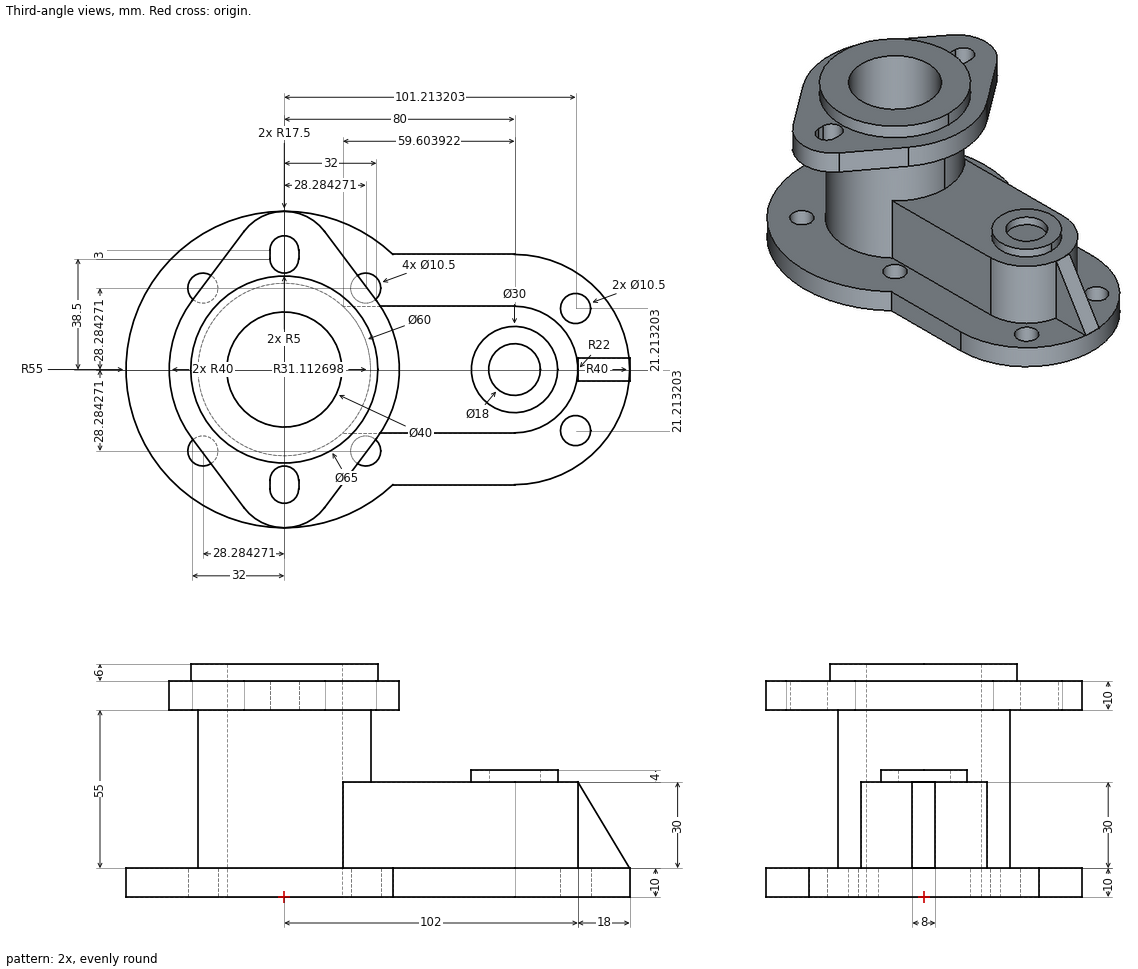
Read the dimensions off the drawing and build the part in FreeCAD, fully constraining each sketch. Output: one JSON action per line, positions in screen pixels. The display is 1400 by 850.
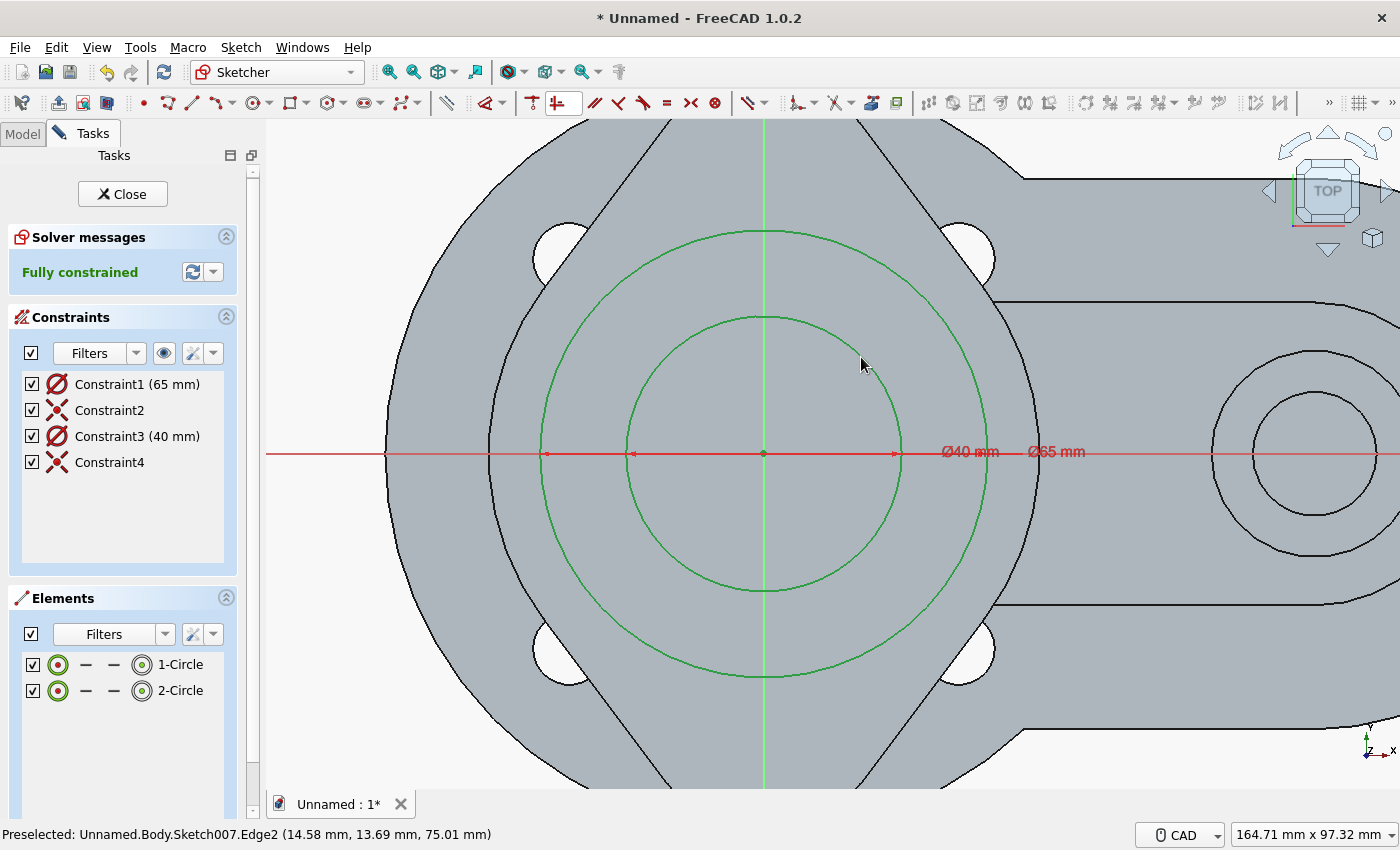
{"action": "left_click", "coordinate": [123, 194]}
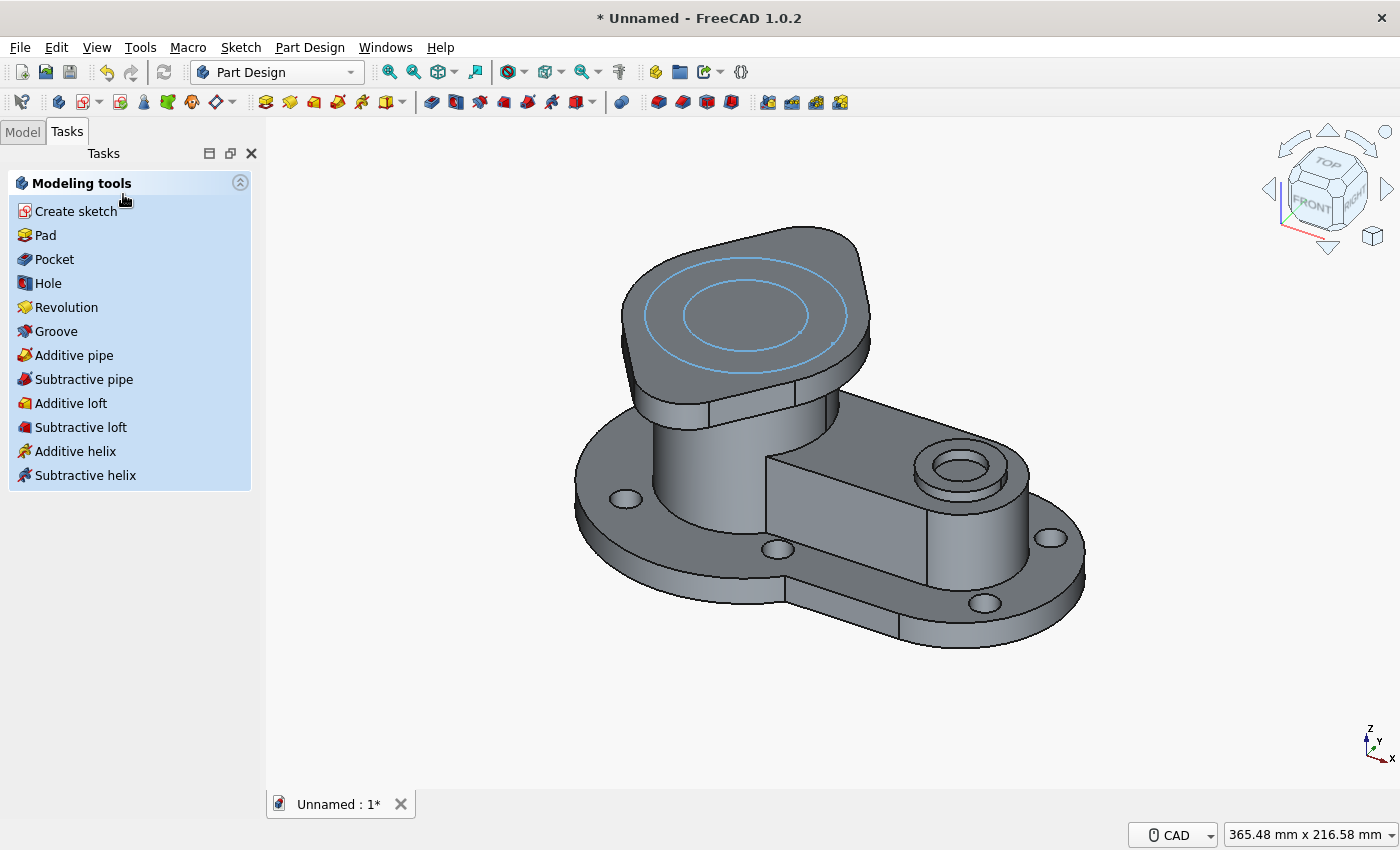
{"action": "left_click", "coordinate": [266, 102]}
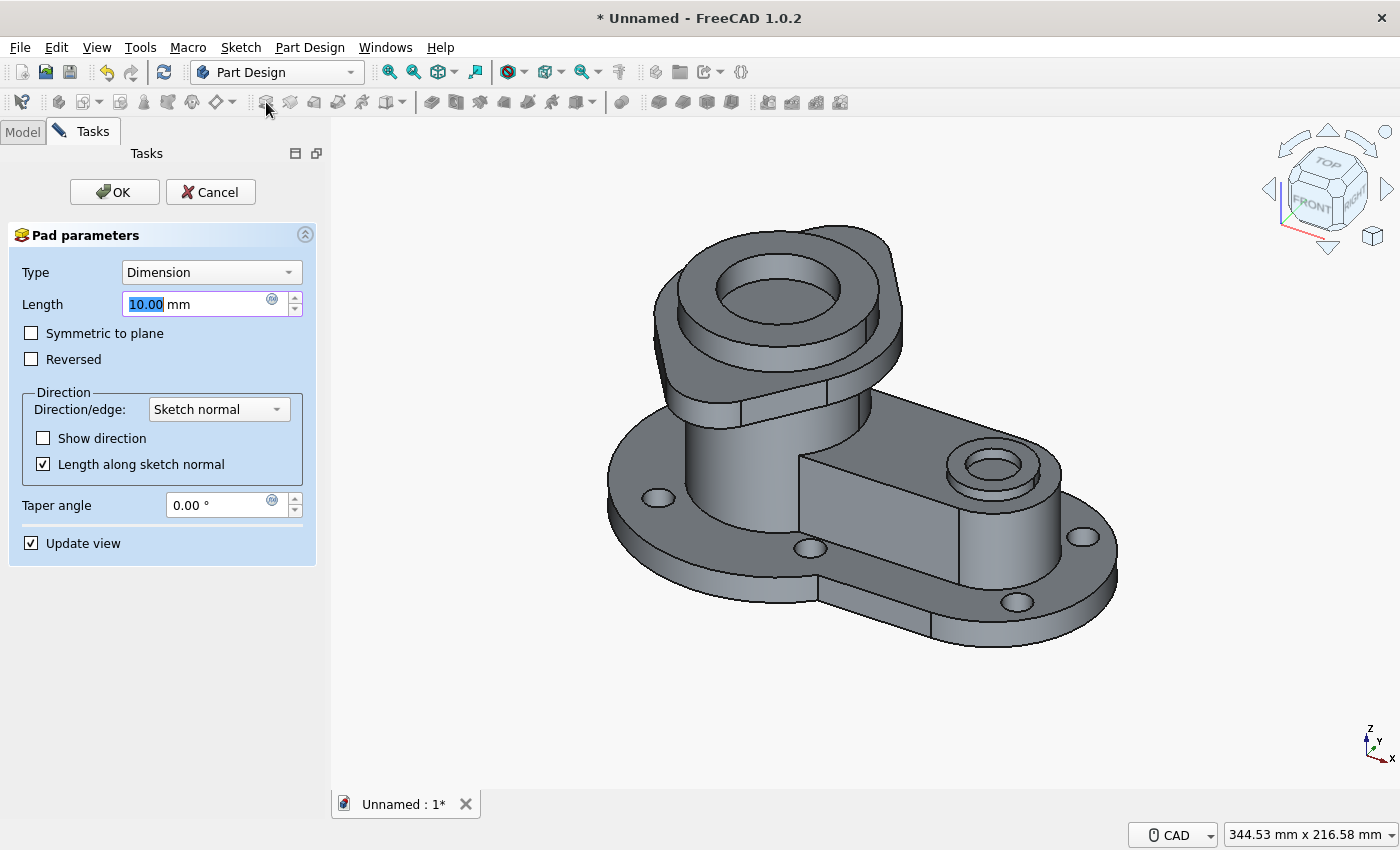
{"action": "type", "text": "6"}
{"action": "key", "text": "Tab"}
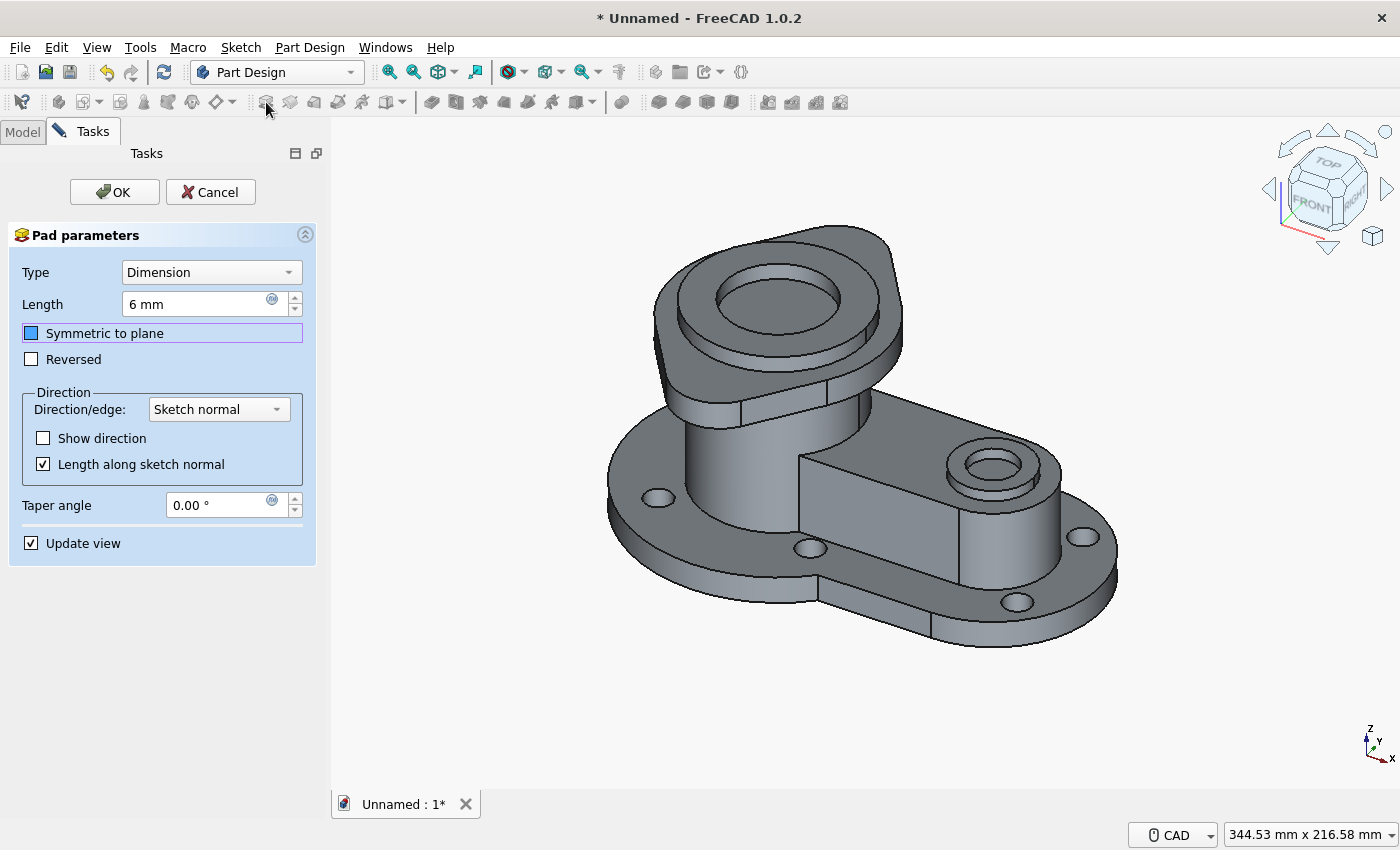
{"action": "left_click", "coordinate": [115, 192]}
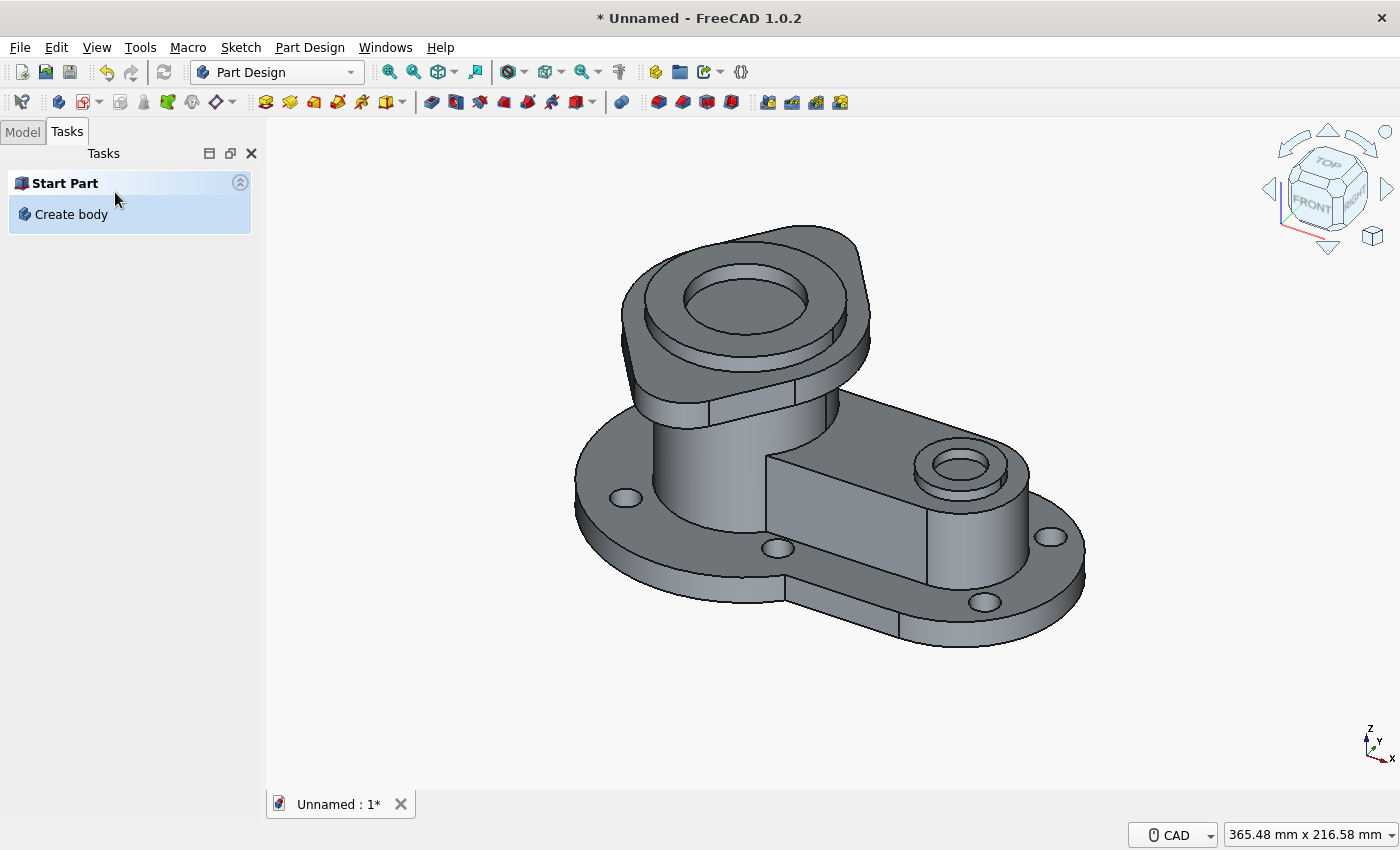
{"action": "left_click", "coordinate": [819, 241]}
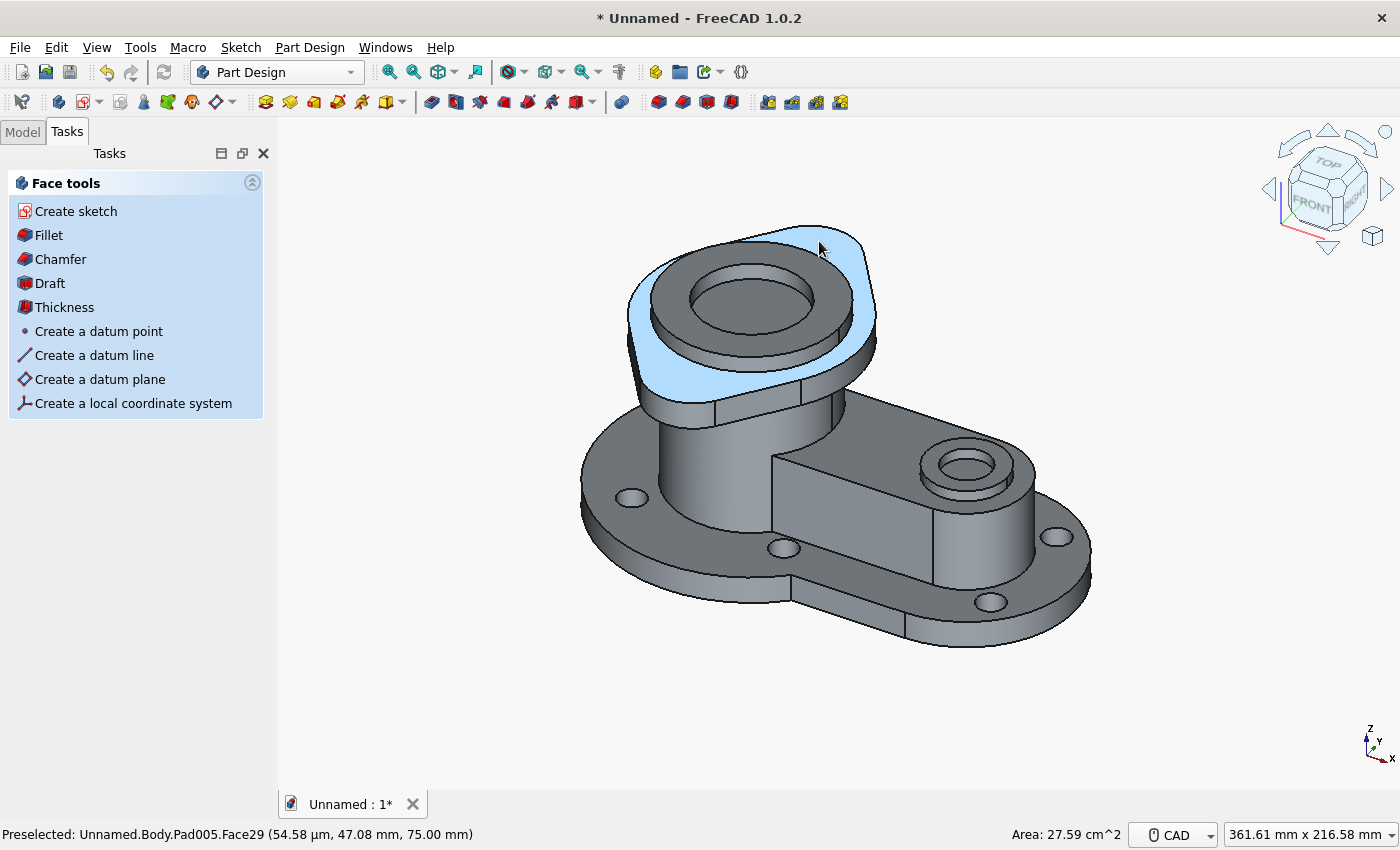
{"action": "left_click", "coordinate": [84, 102]}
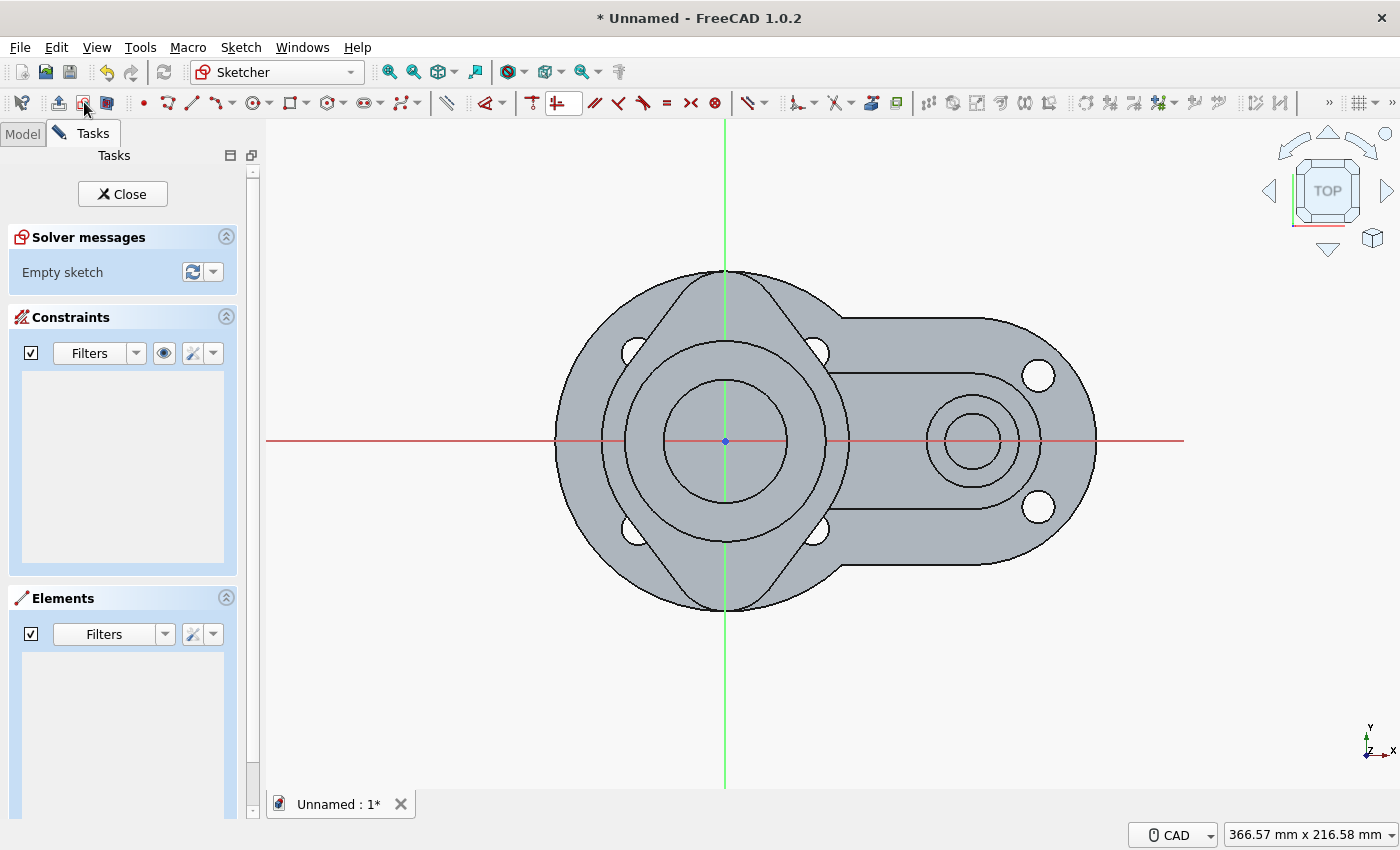
{"action": "scroll", "coordinate": [708, 436], "scroll_direction": "up", "scroll_amount": 6}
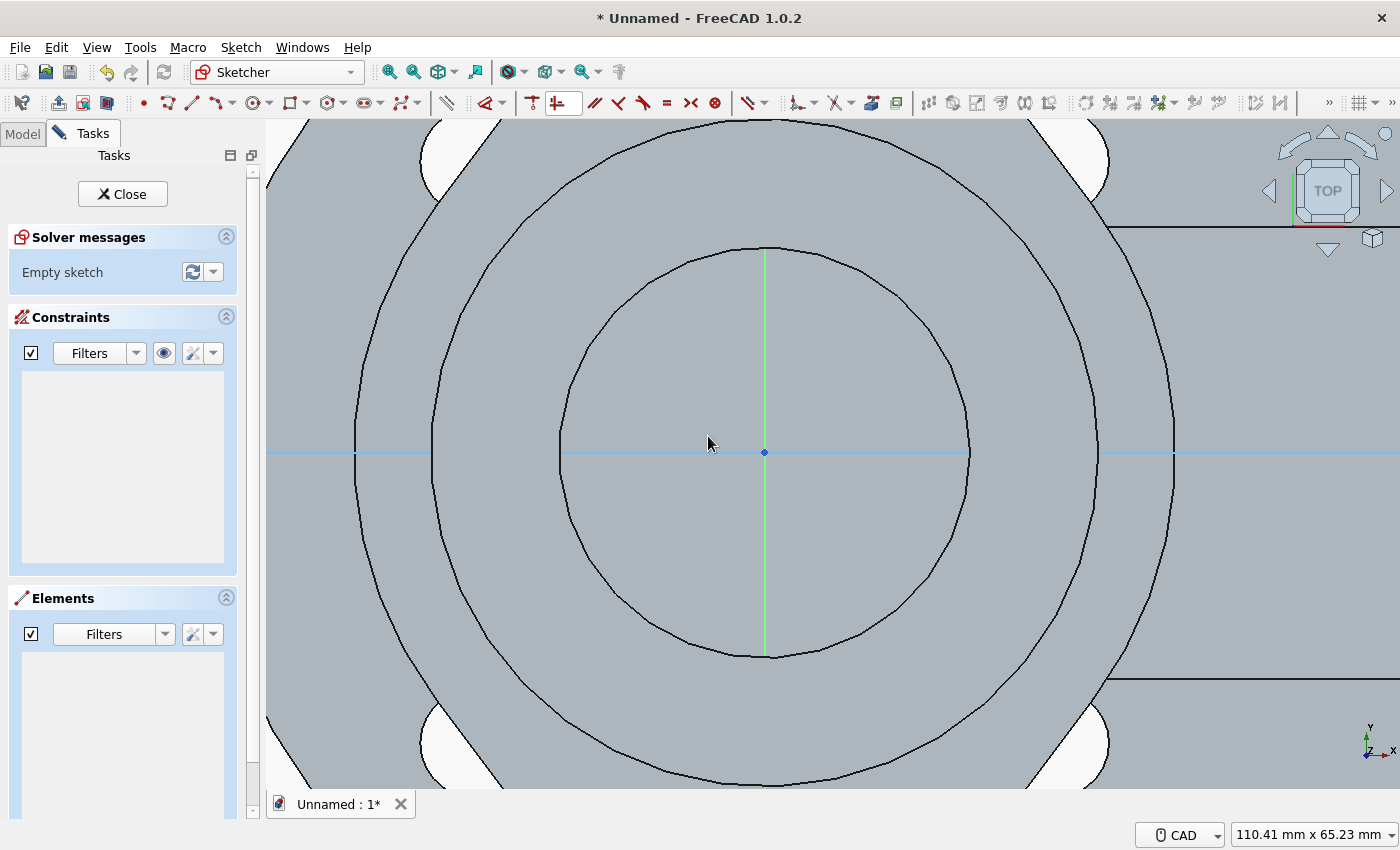
{"action": "key", "text": "g c"}